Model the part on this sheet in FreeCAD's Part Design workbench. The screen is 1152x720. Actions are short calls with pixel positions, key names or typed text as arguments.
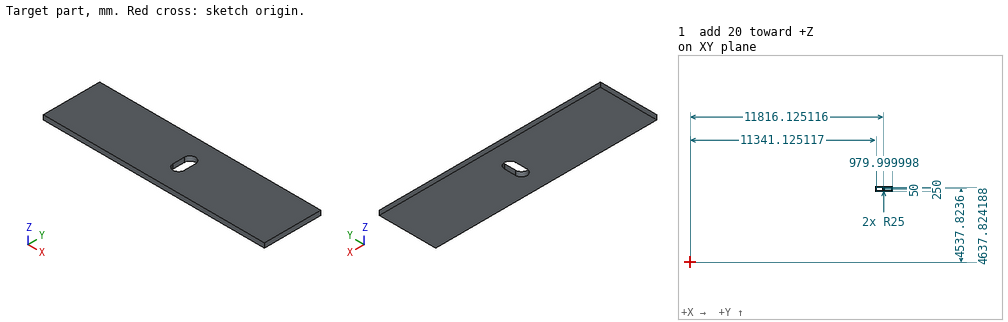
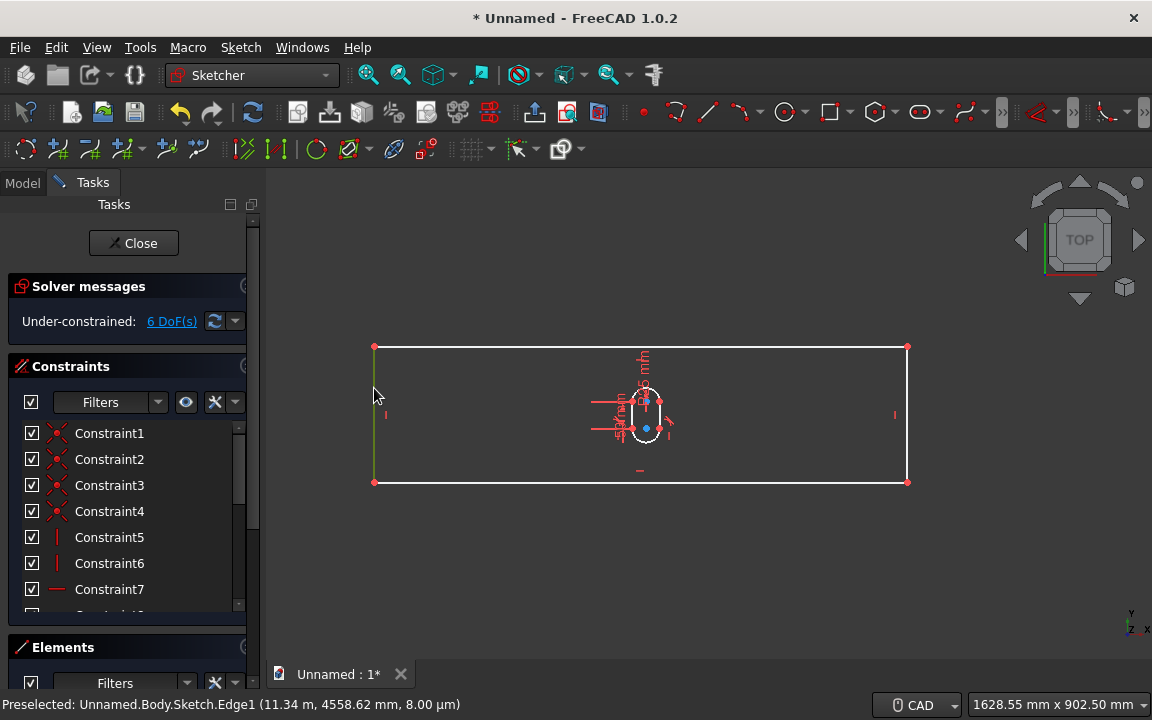
key(i)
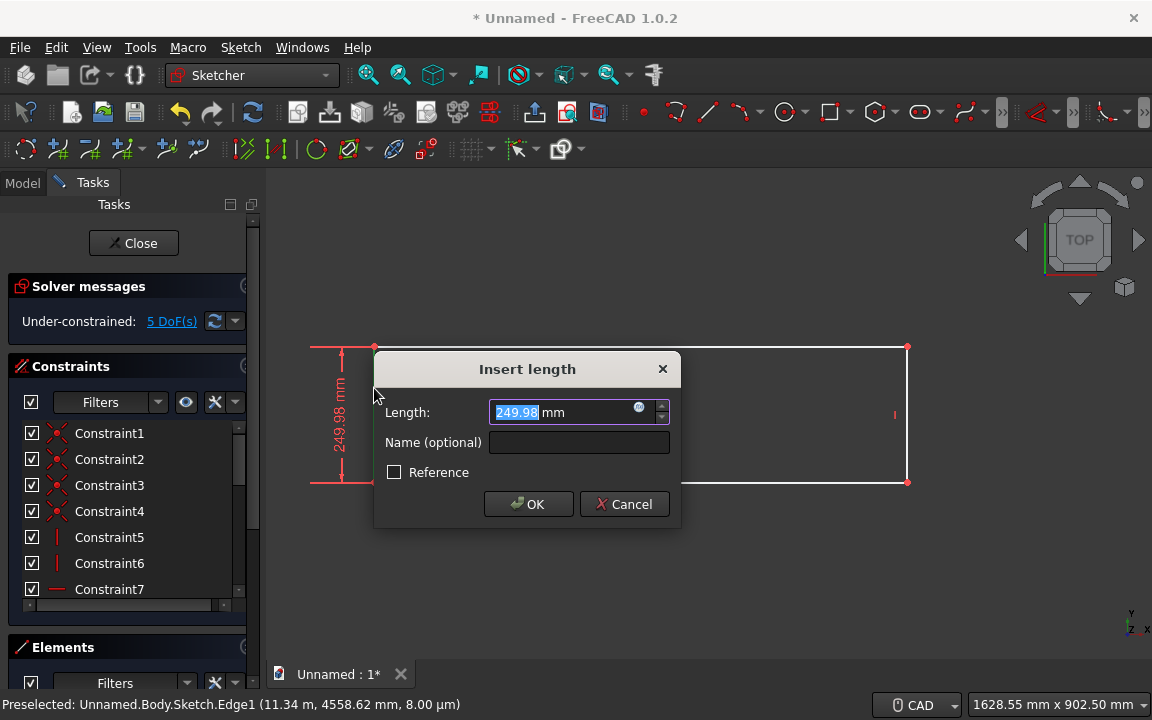
text(250)
key(Return)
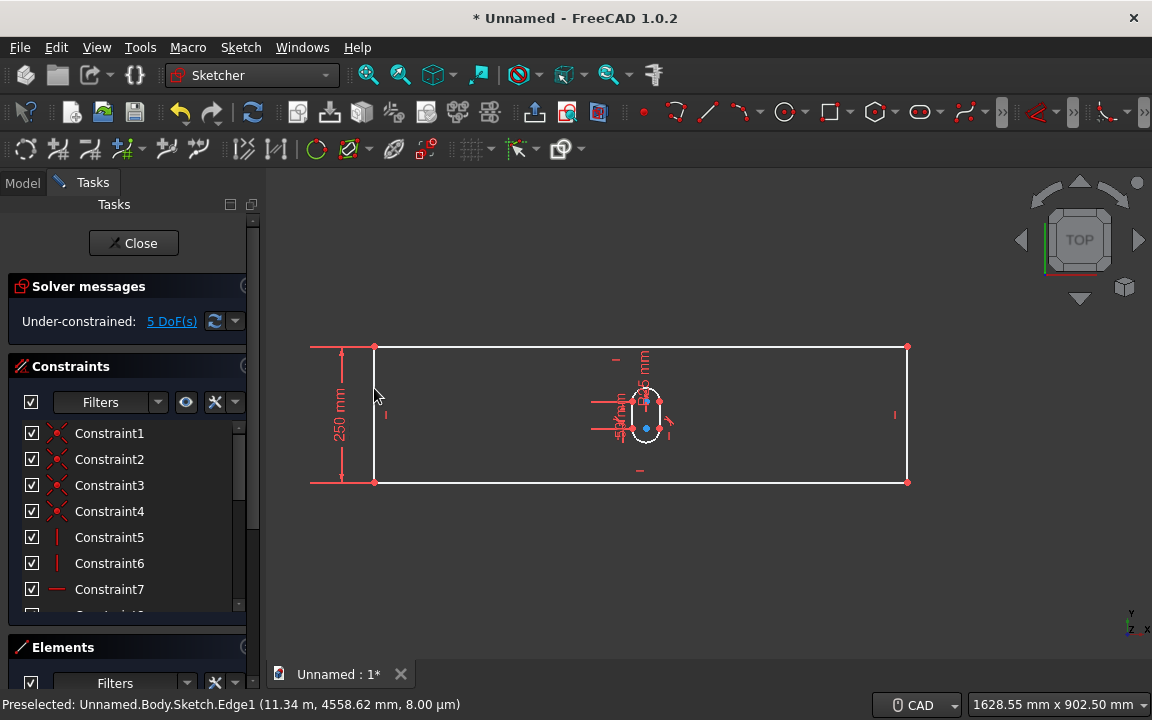
click(534, 483)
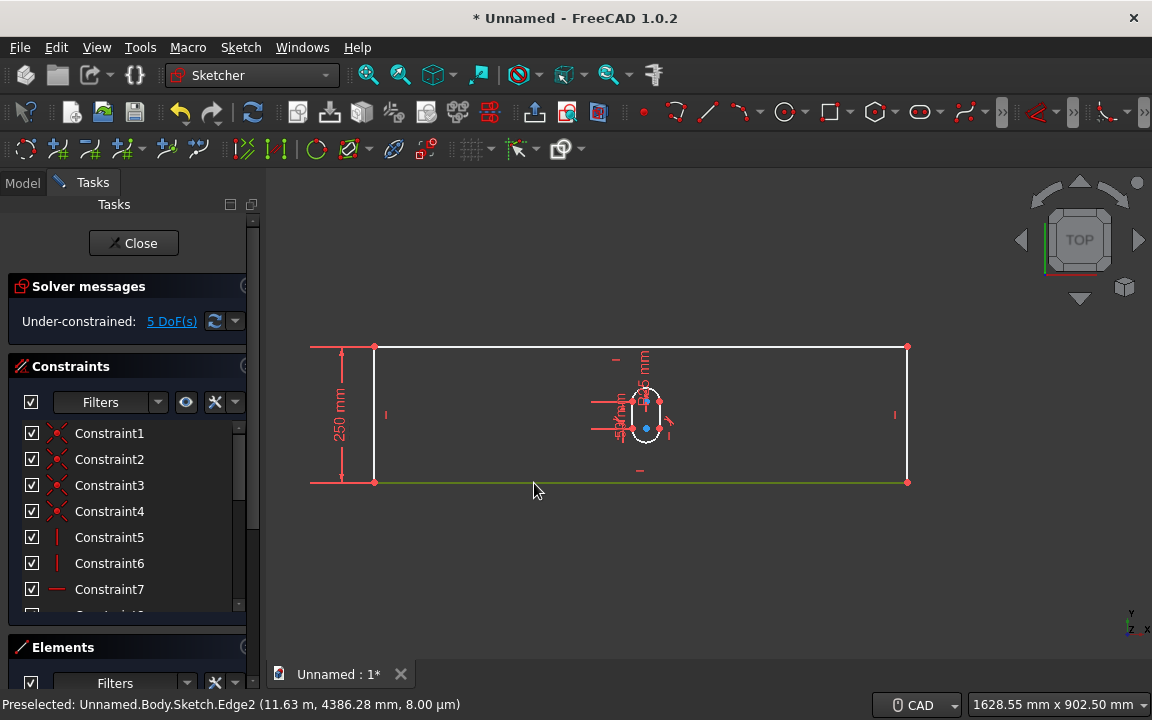
key(l)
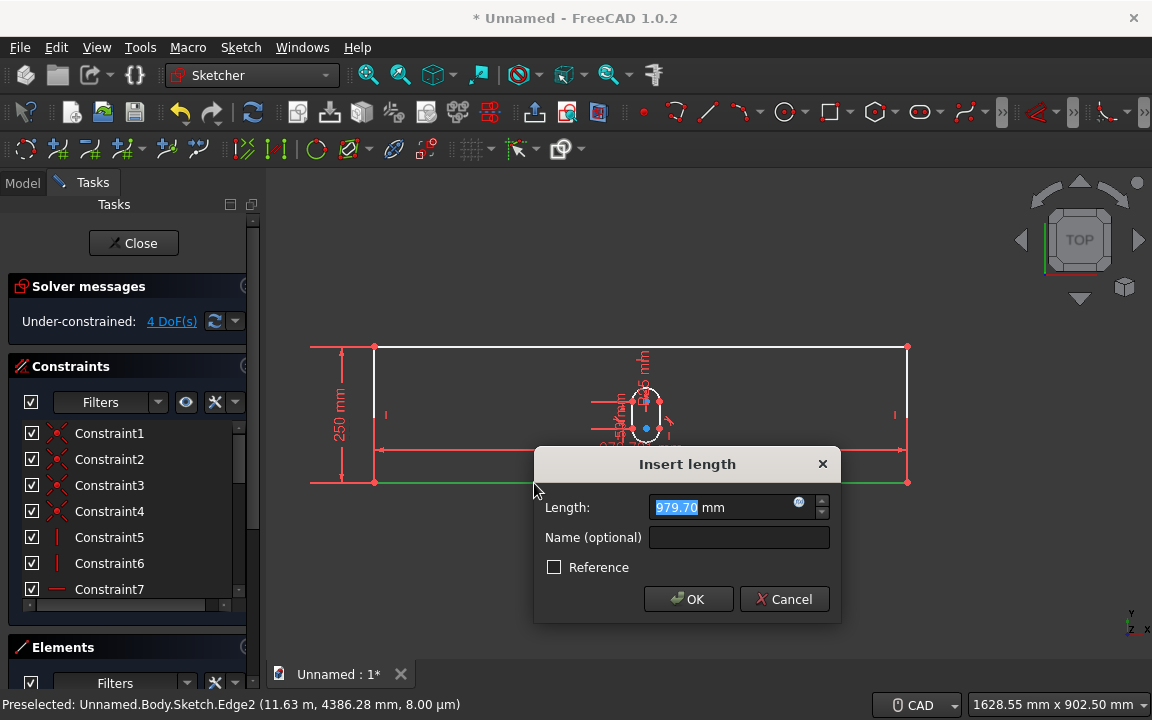
text(979.999998)
key(Return)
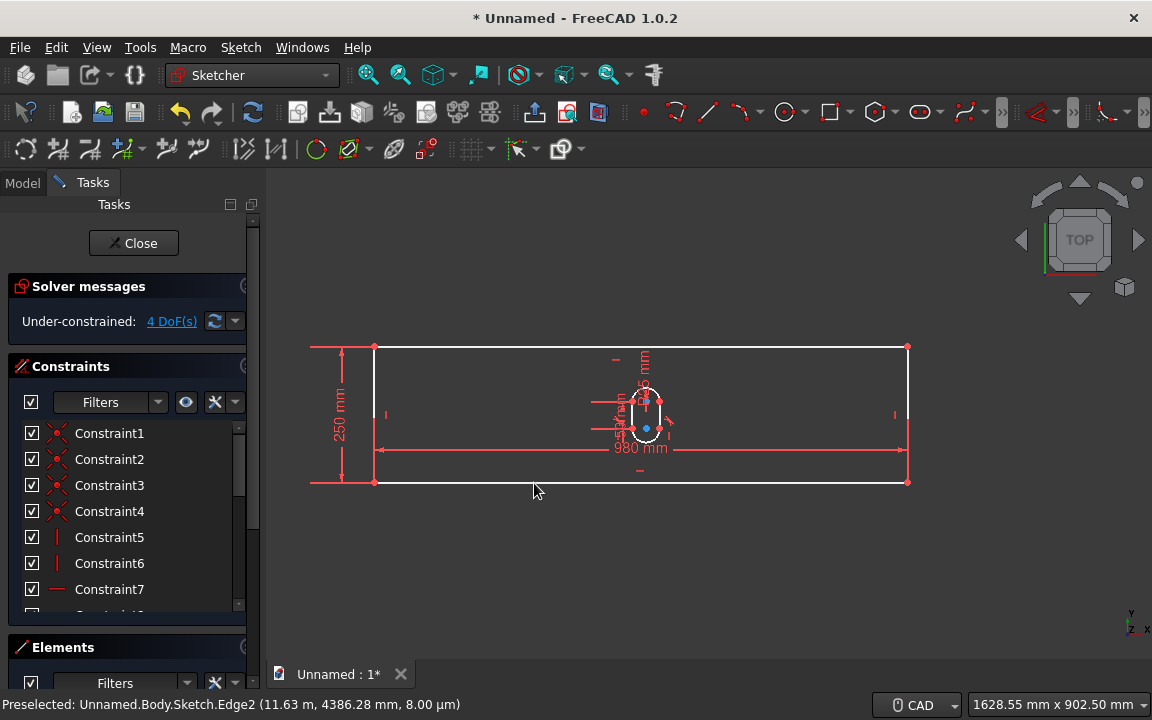
click(660, 402)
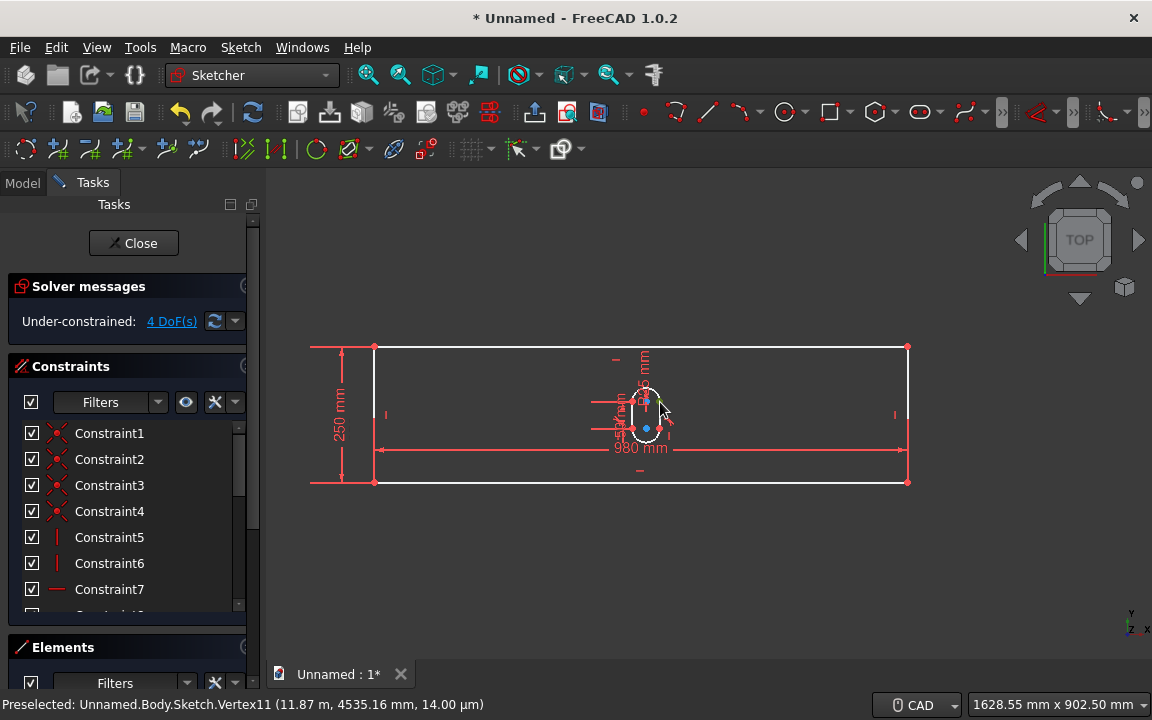
click(1058, 112)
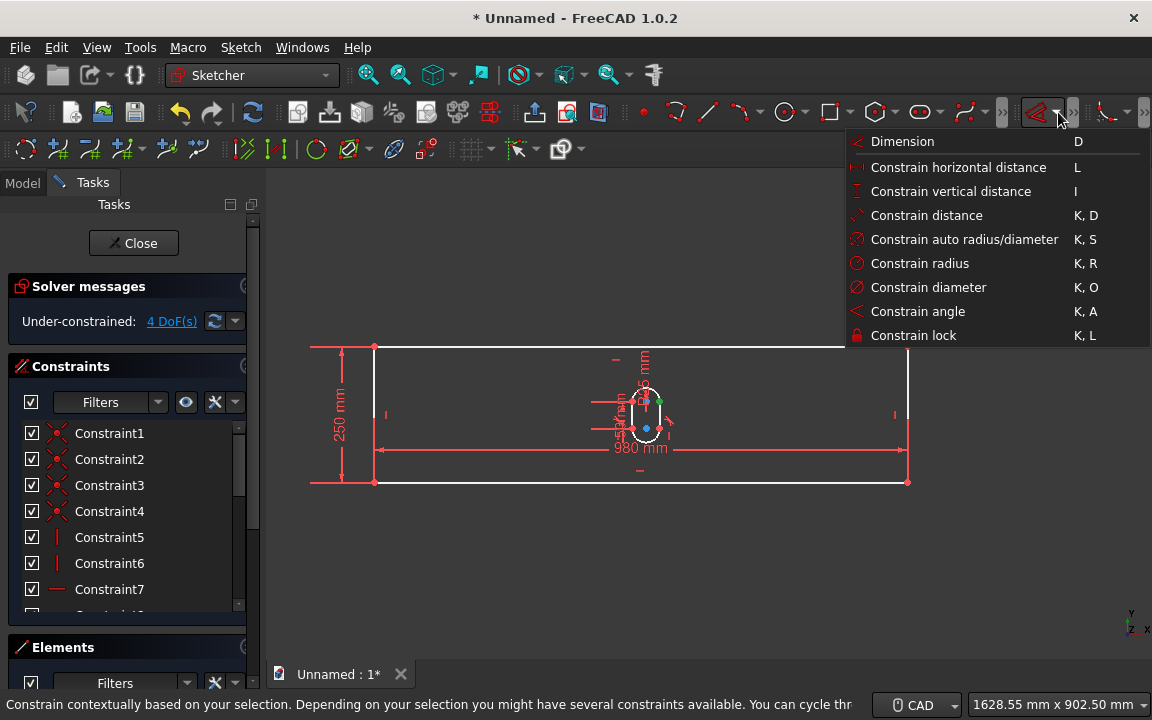
click(998, 191)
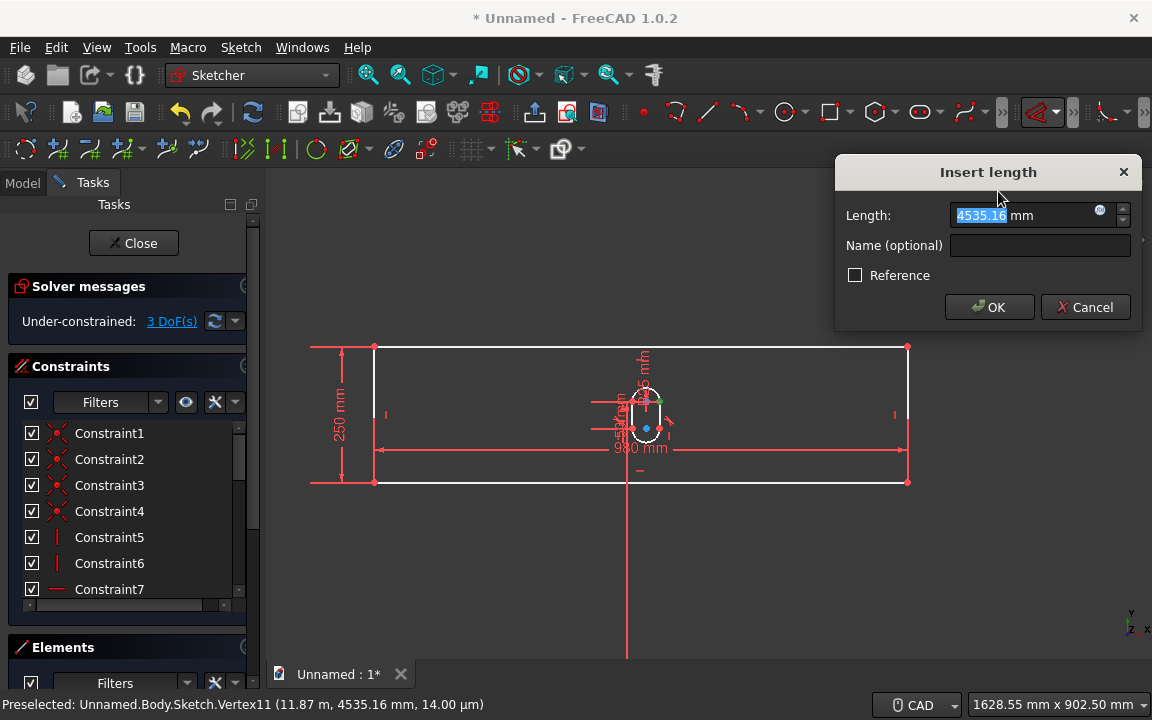
text(4537.8236)
key(Return)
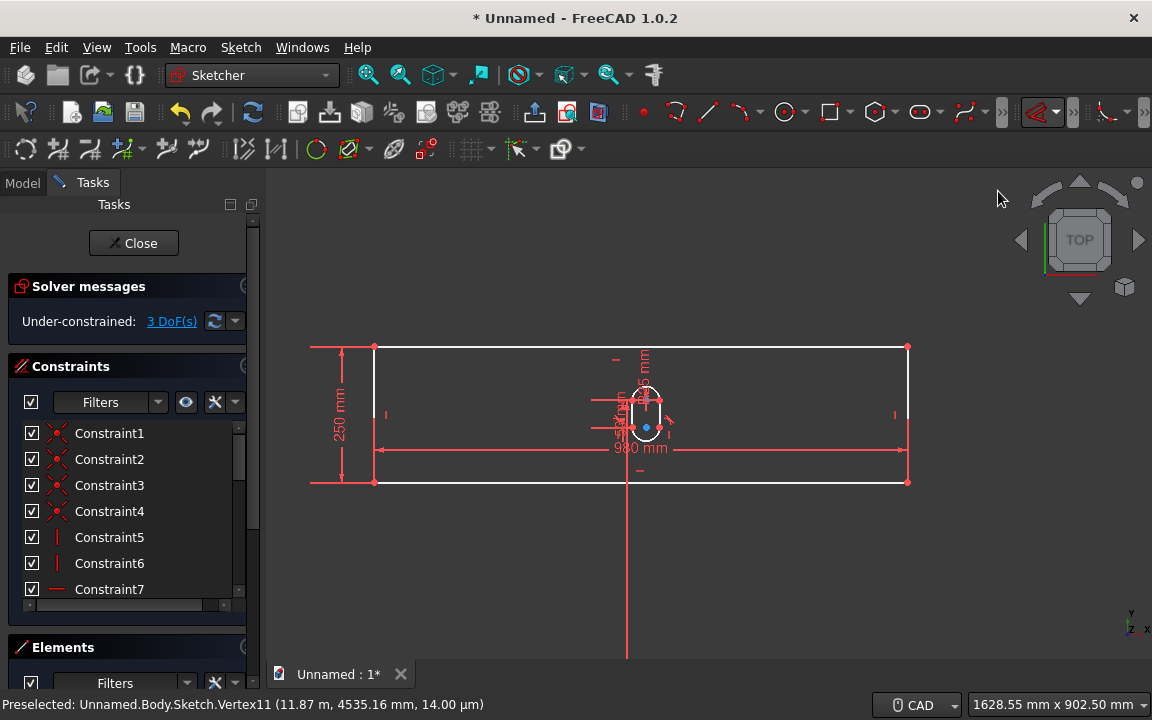
click(374, 347)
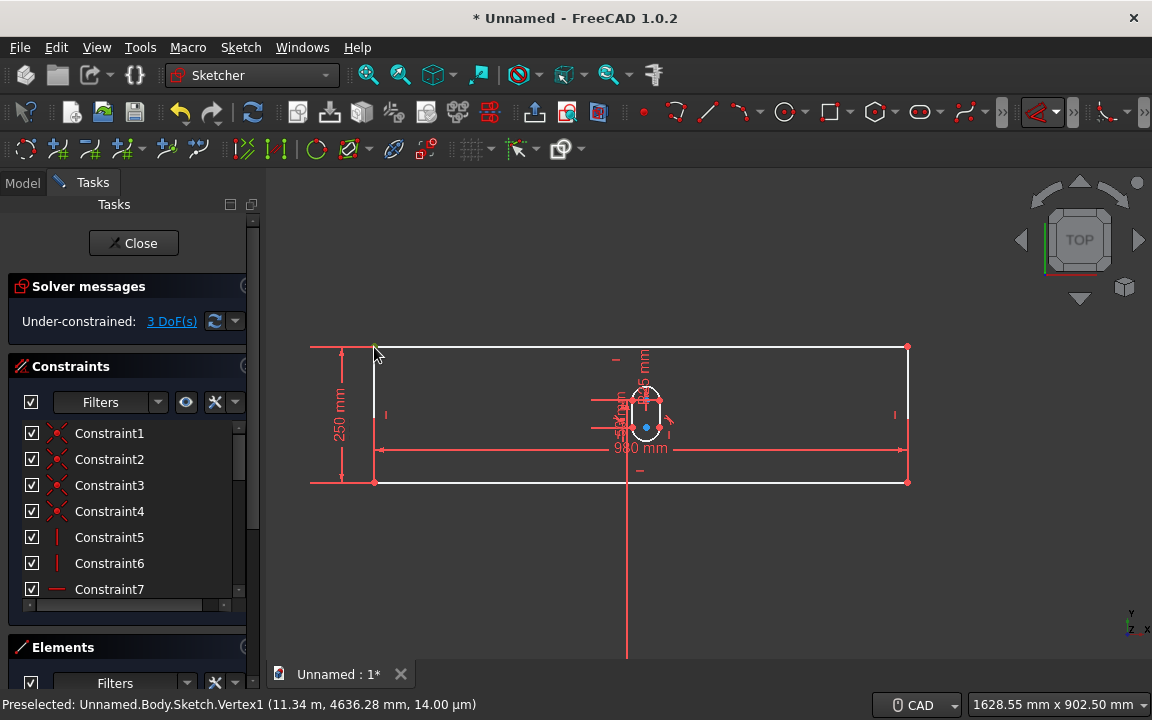
key(i)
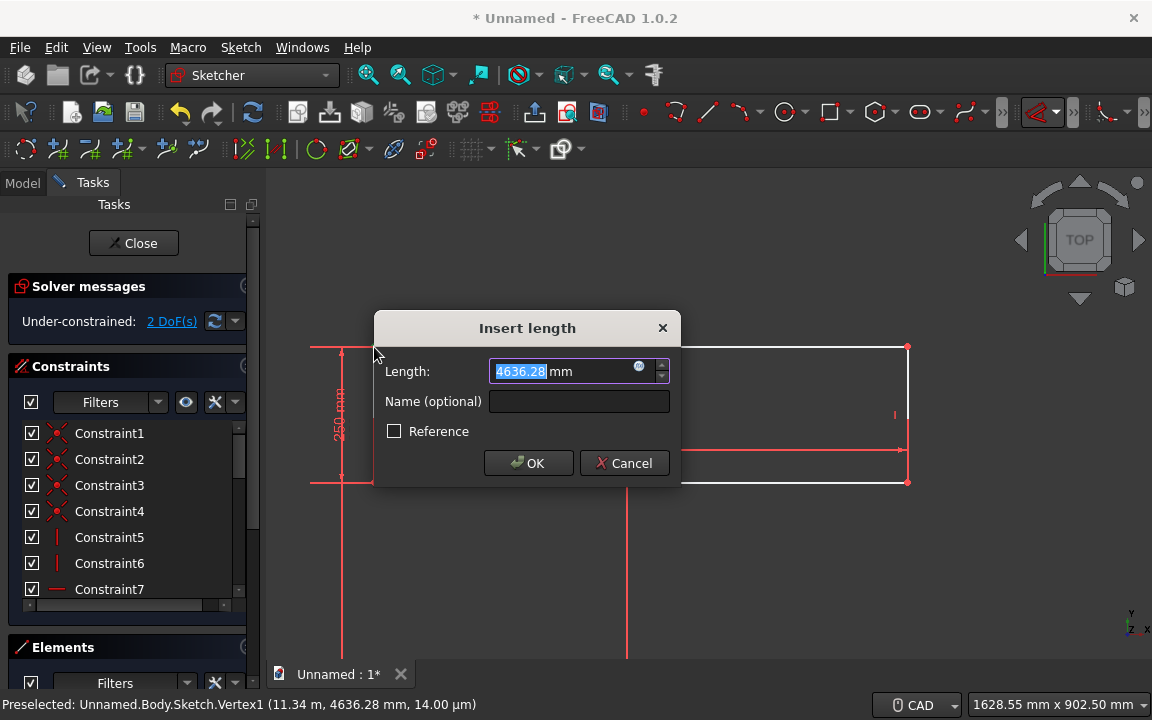
text(4637.824188)
key(Return)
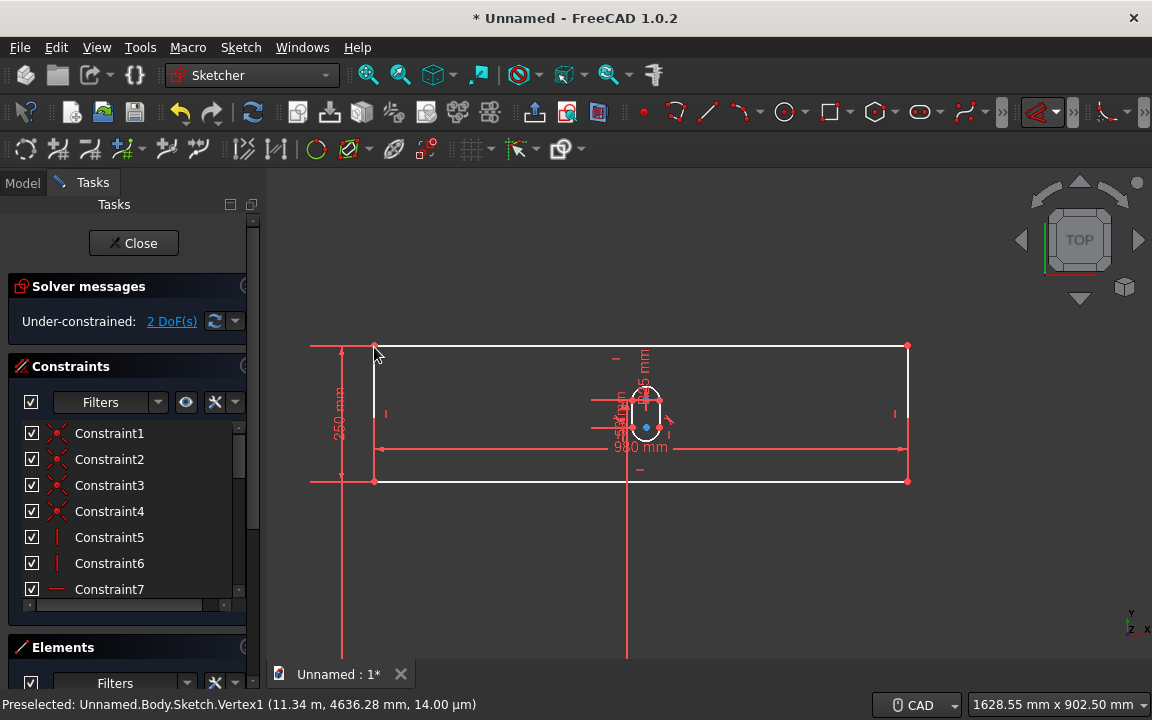
click(374, 346)